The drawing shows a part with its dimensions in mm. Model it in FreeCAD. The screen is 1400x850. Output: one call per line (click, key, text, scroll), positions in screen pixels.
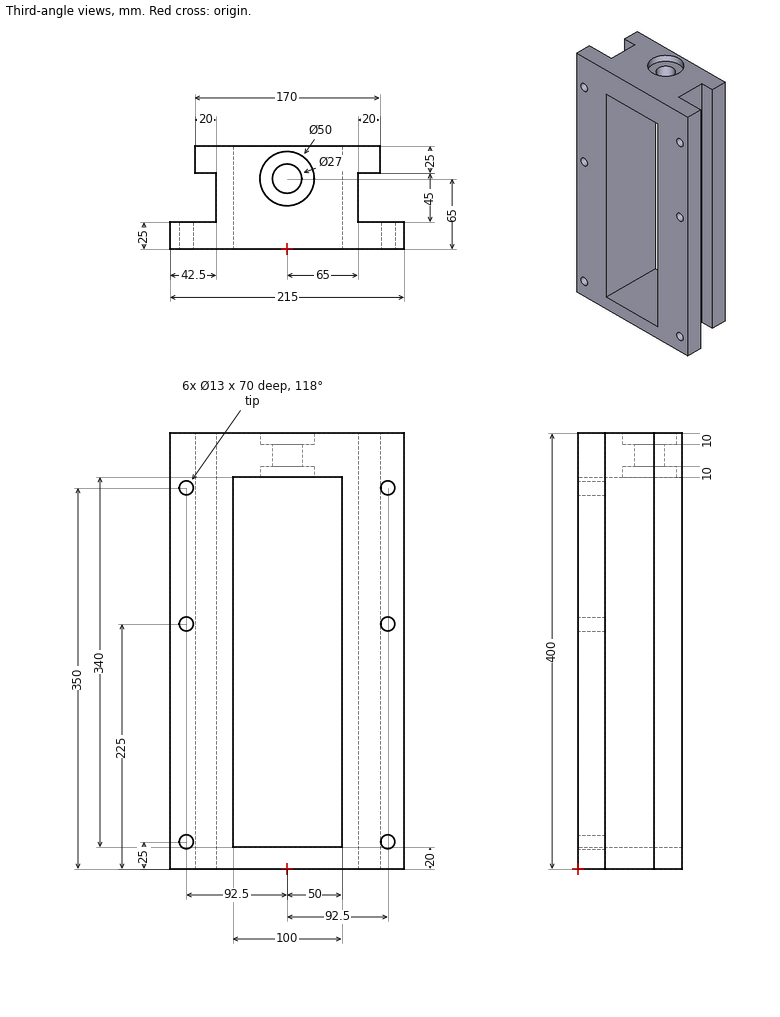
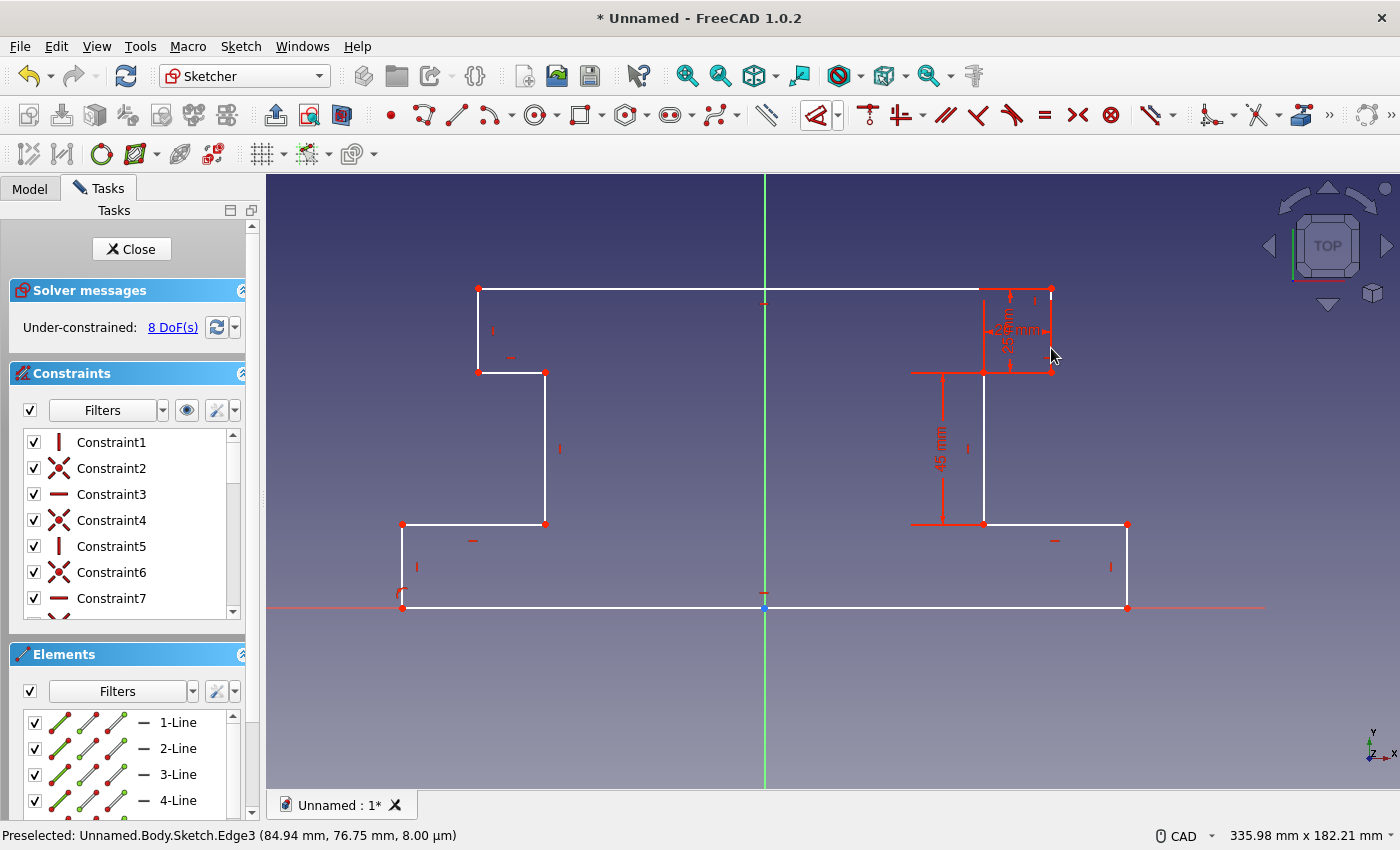
click(478, 314)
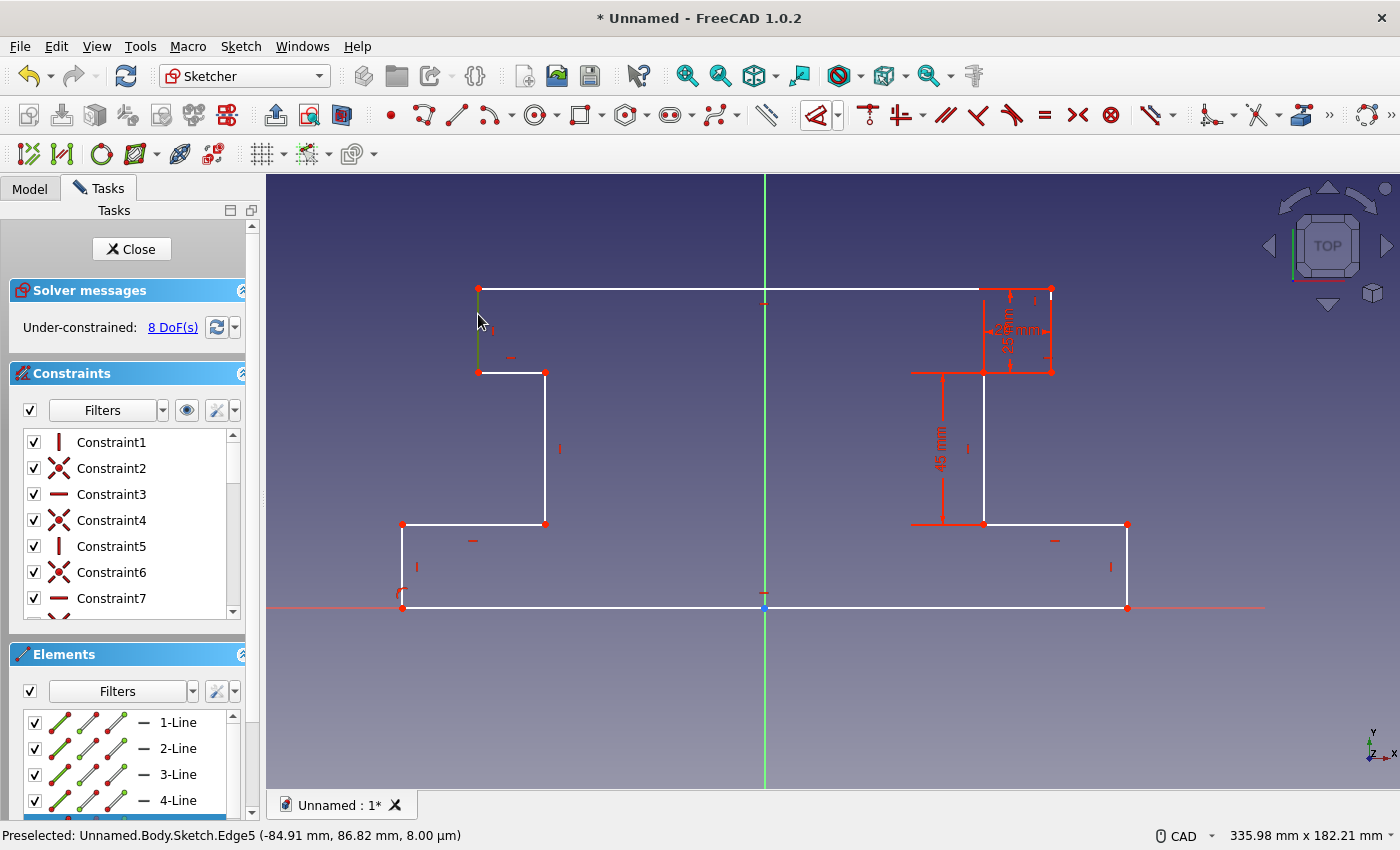
key(i)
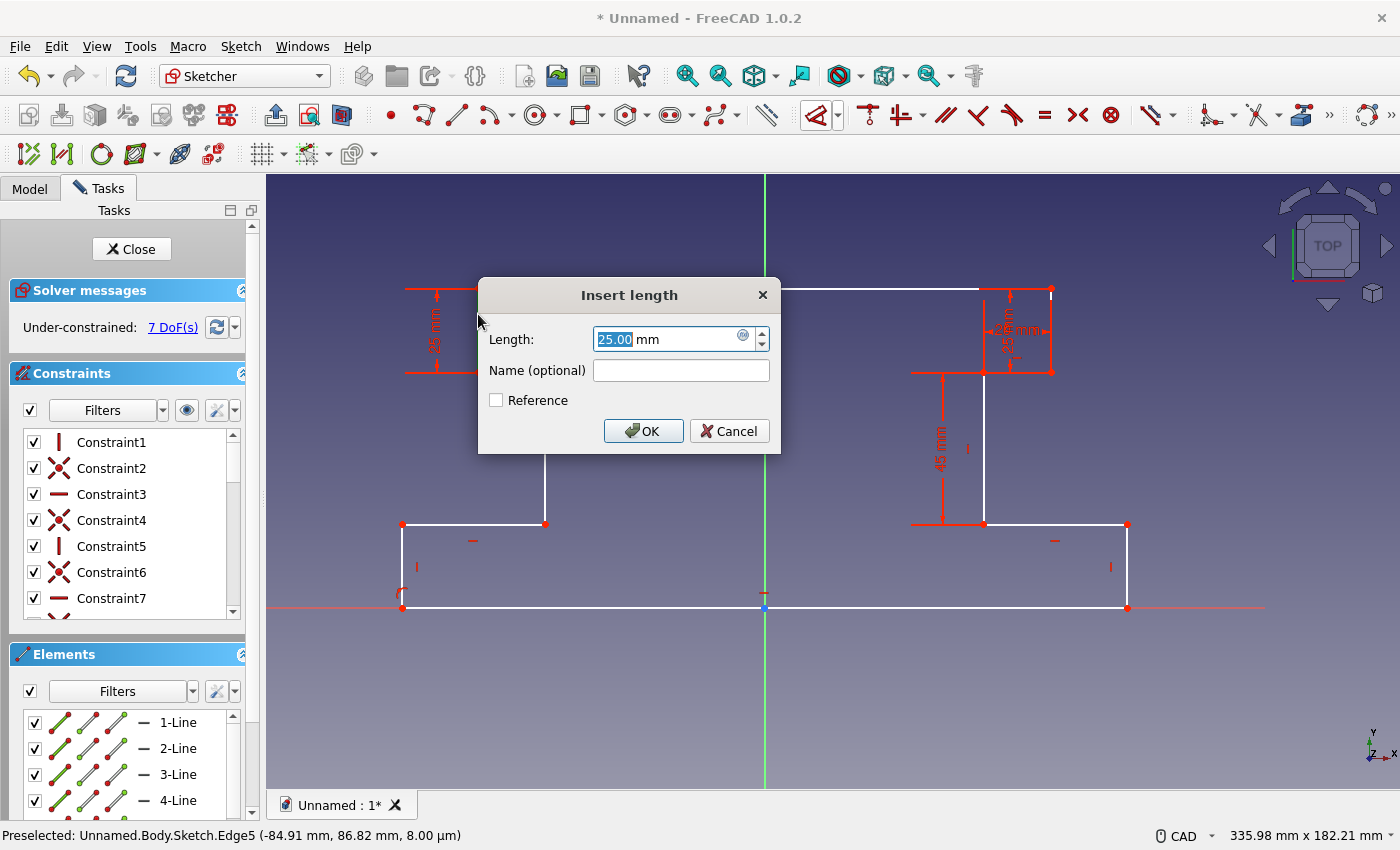
text(25)
key(Return)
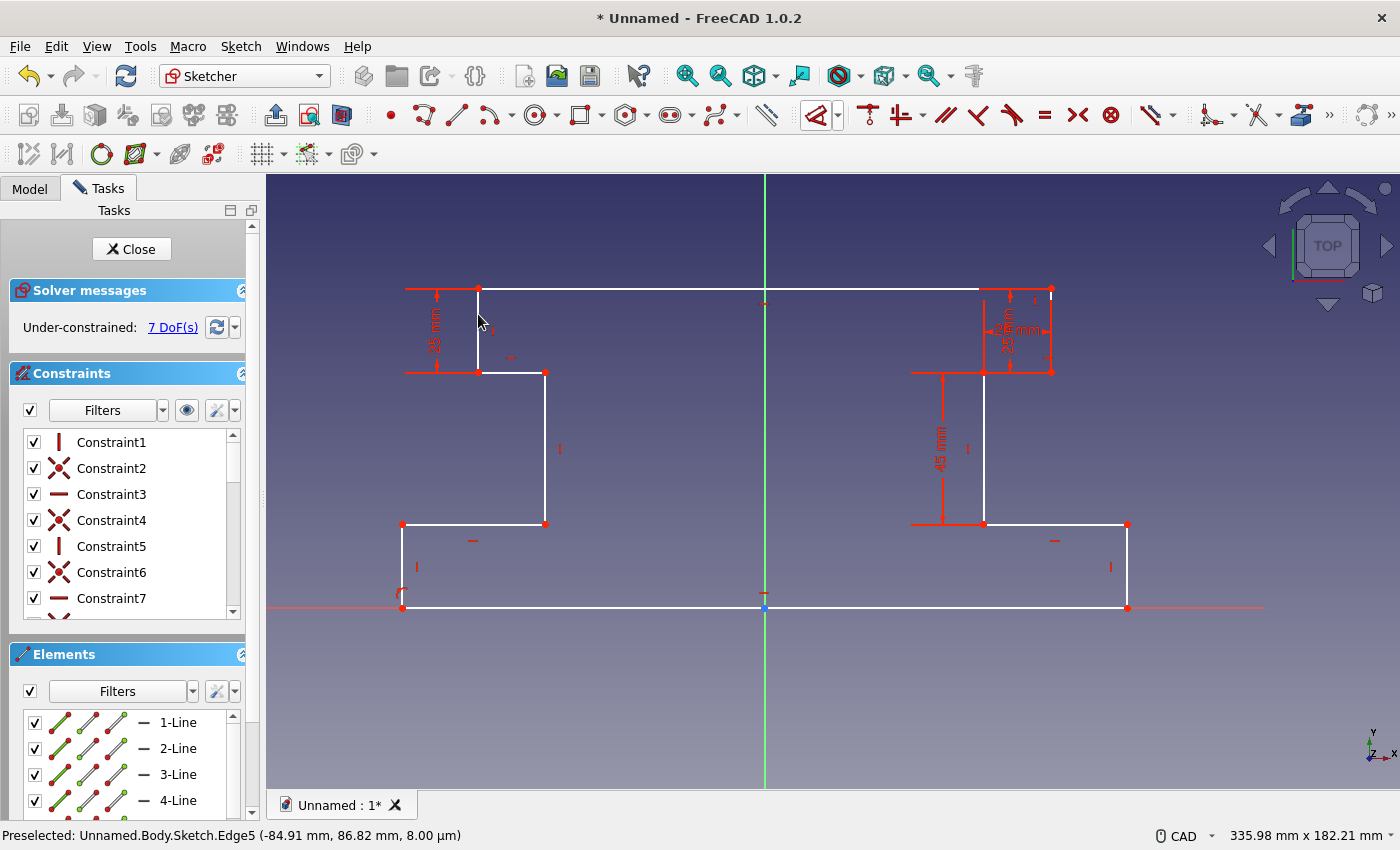
click(498, 373)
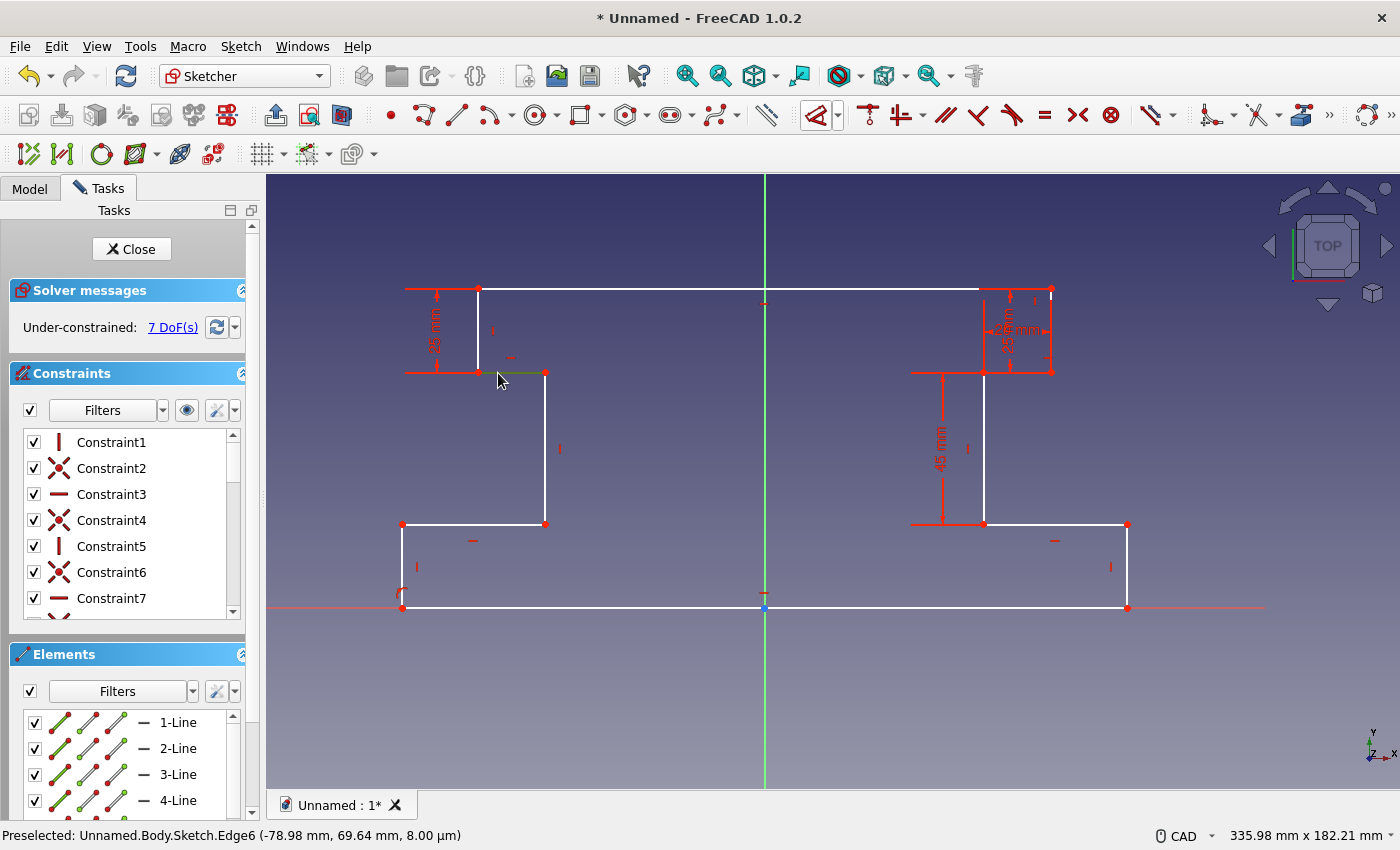
key(l)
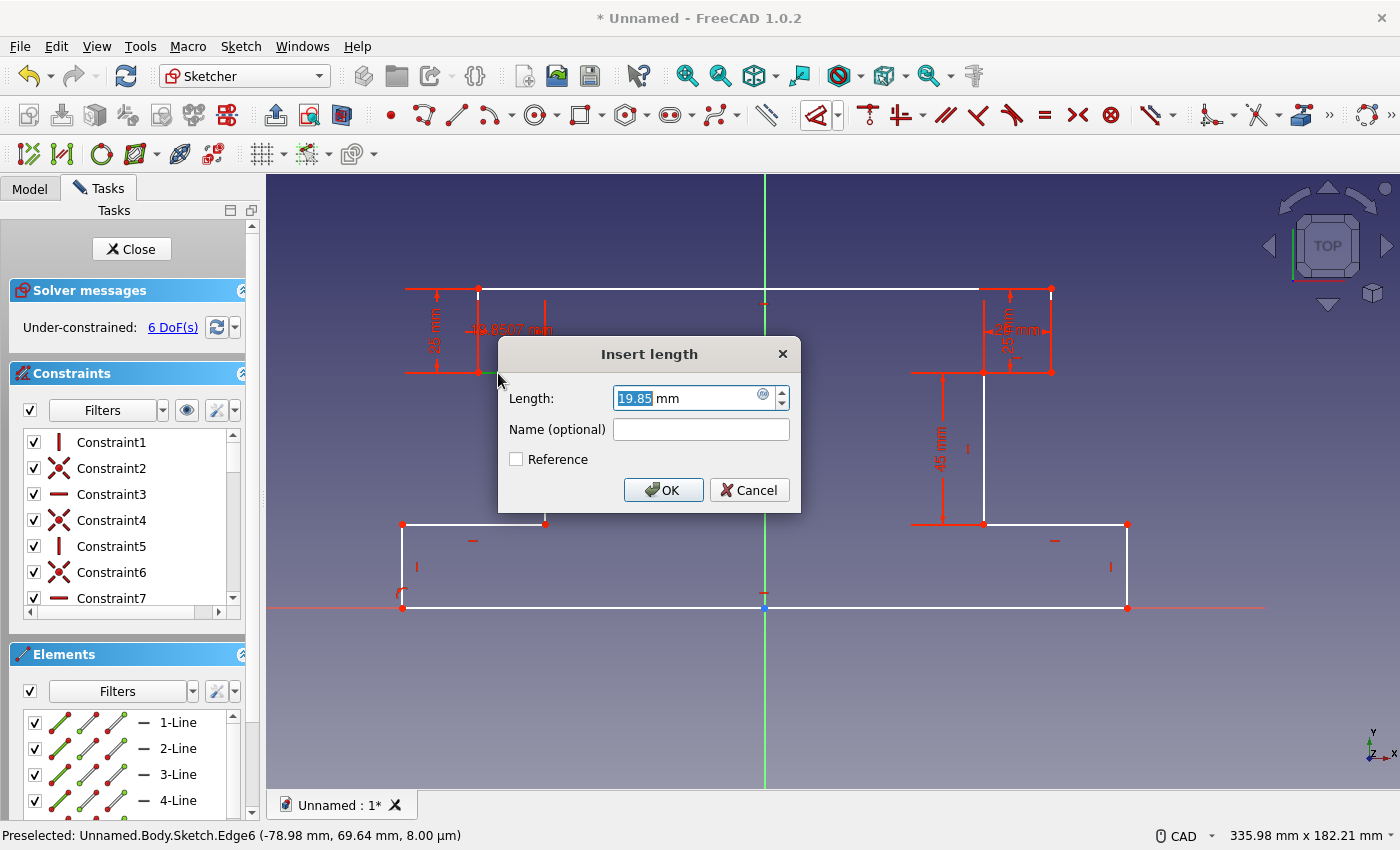
text(20)
key(Return)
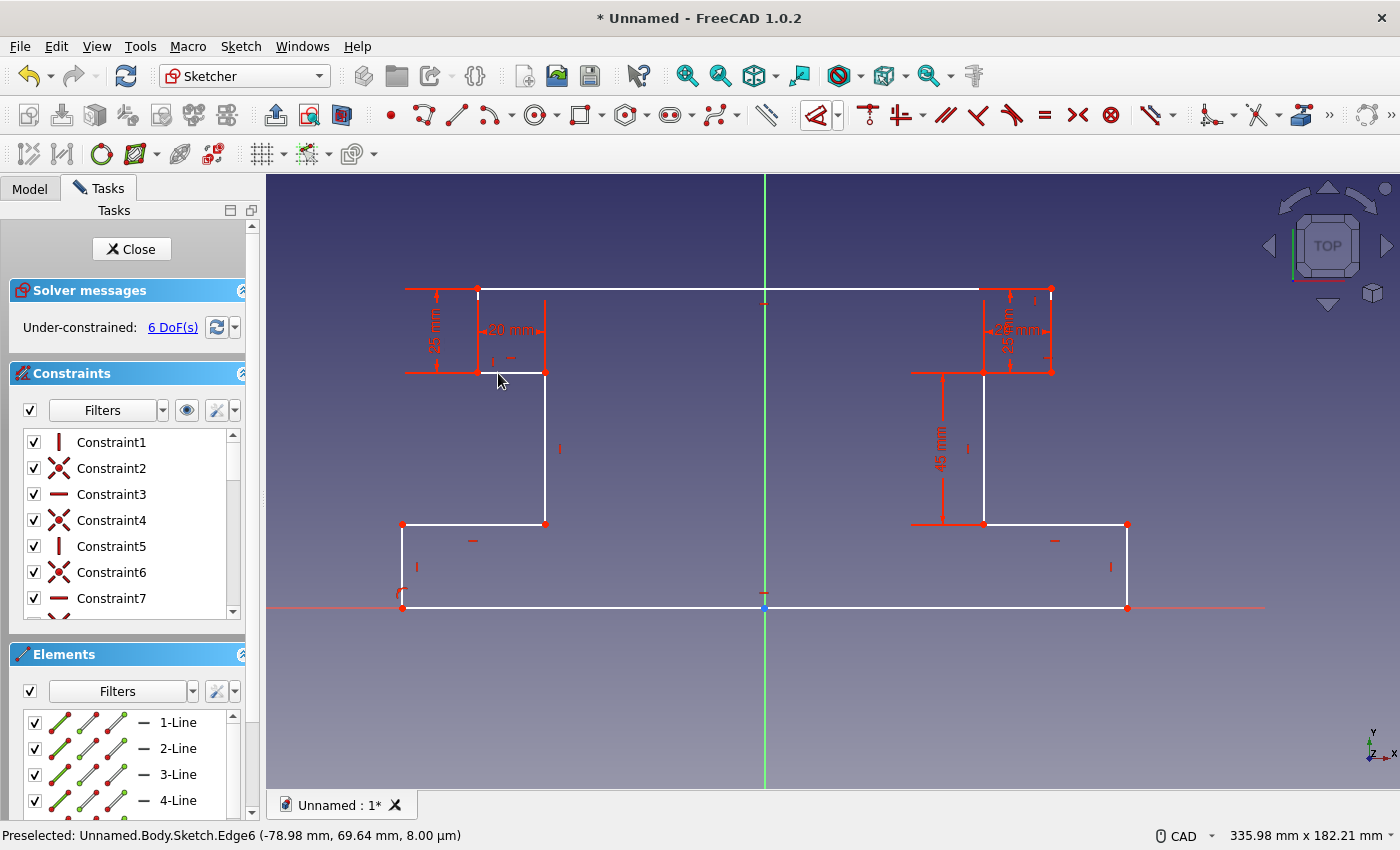
click(545, 419)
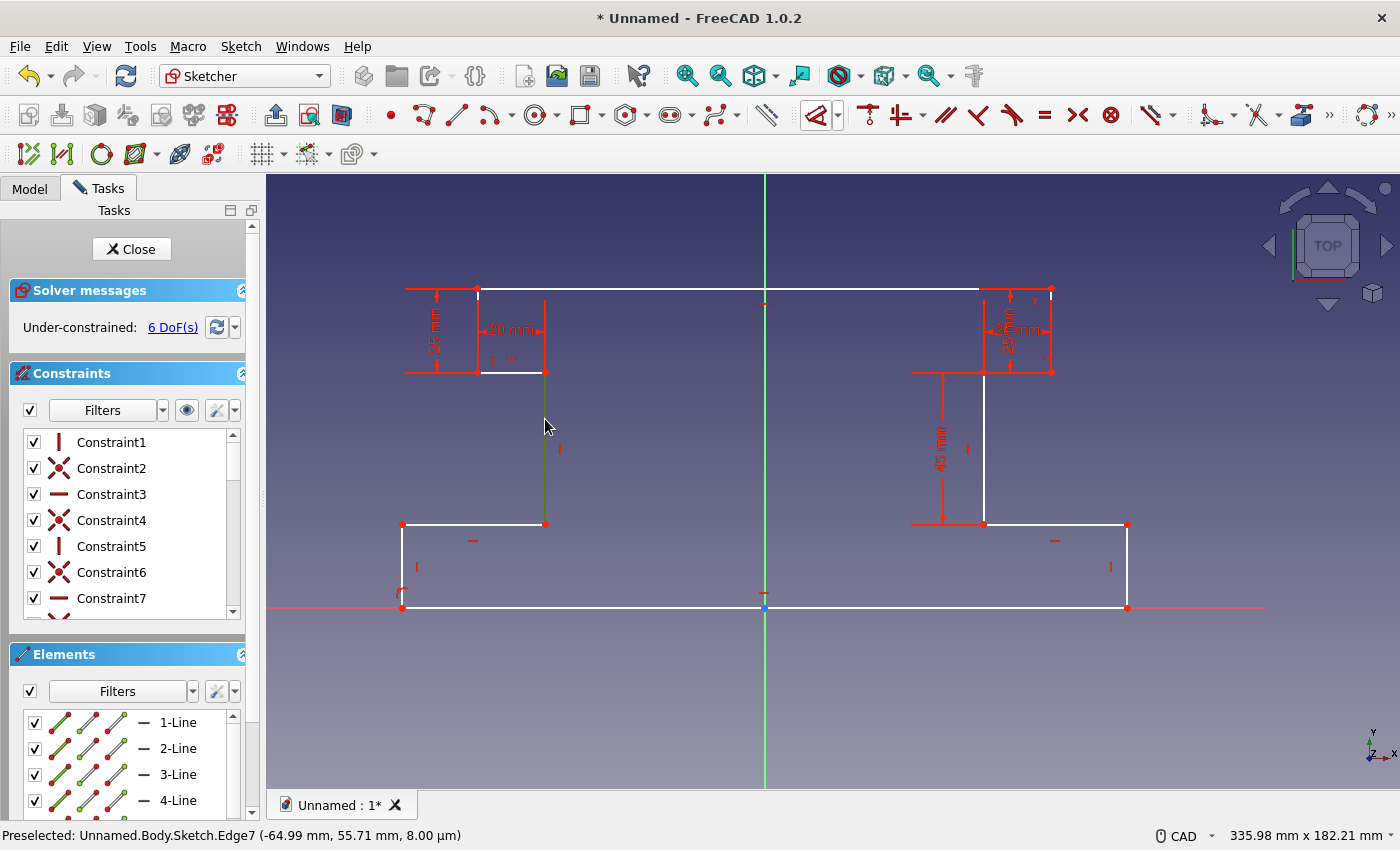
key(i)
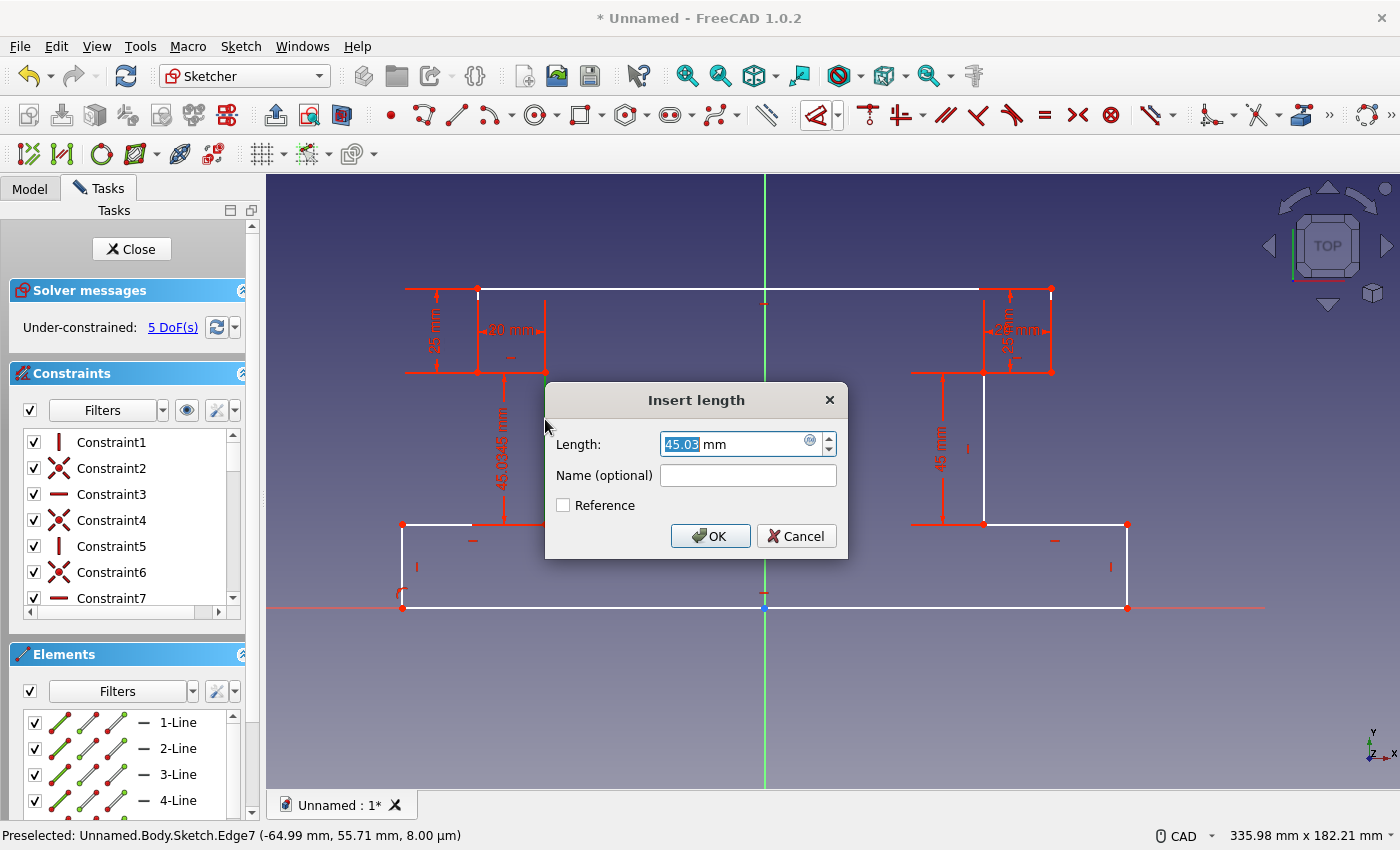
text(45)
key(Return)